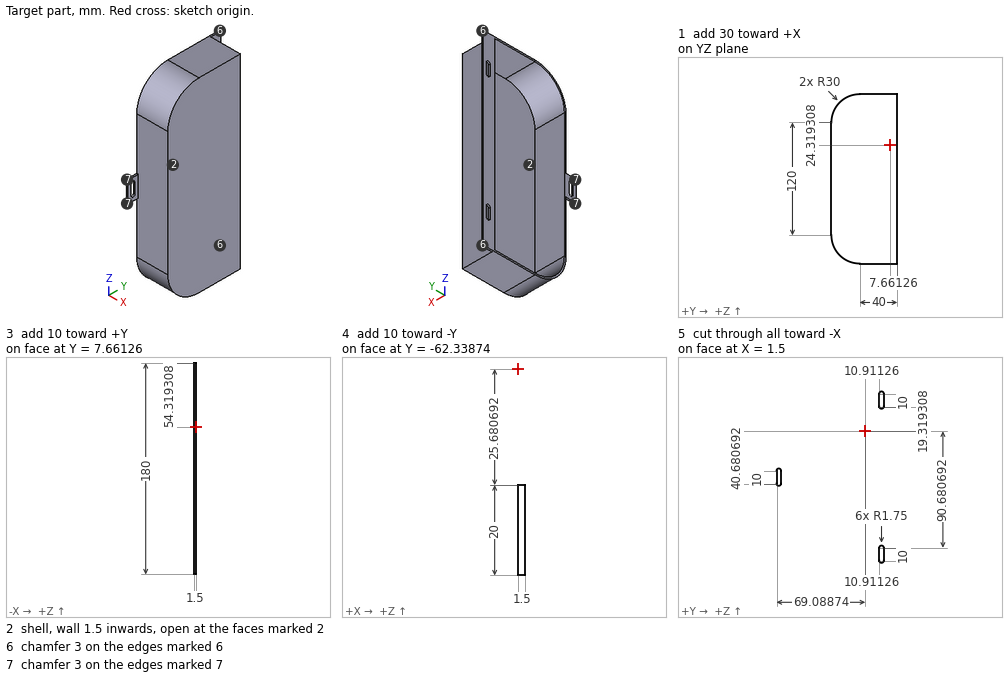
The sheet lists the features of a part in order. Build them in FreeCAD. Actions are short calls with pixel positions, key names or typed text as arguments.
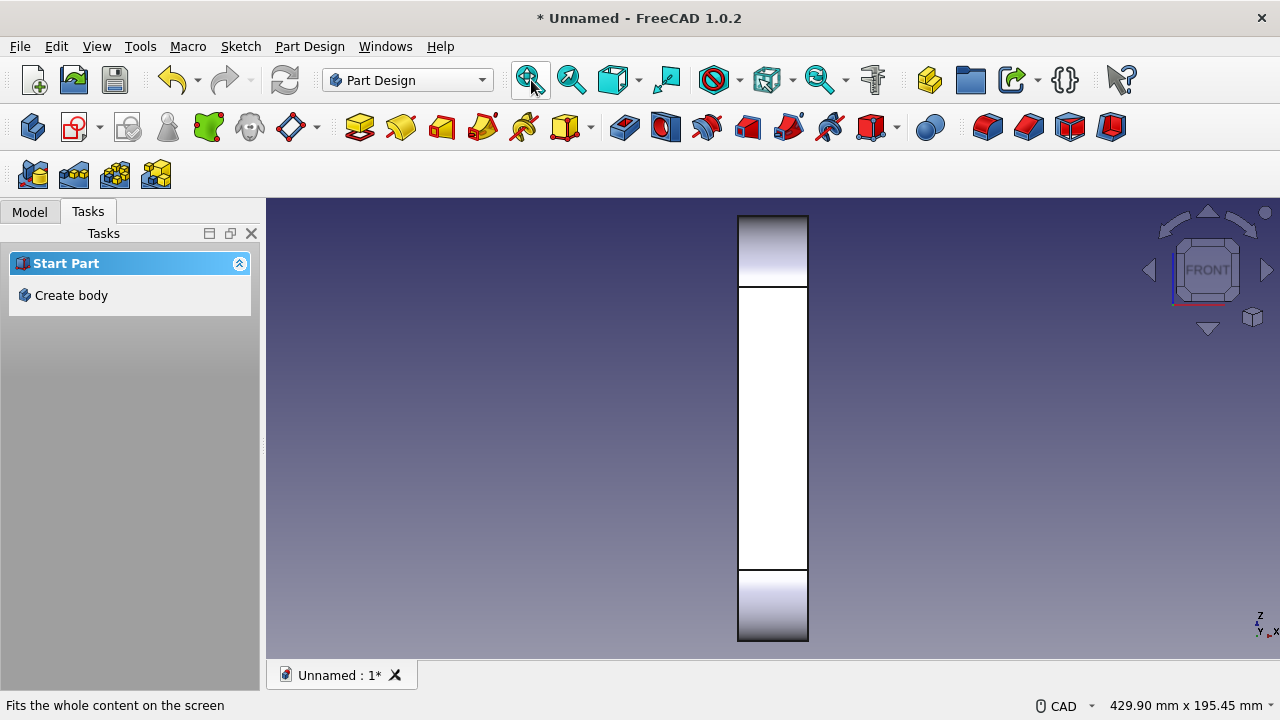
key(3)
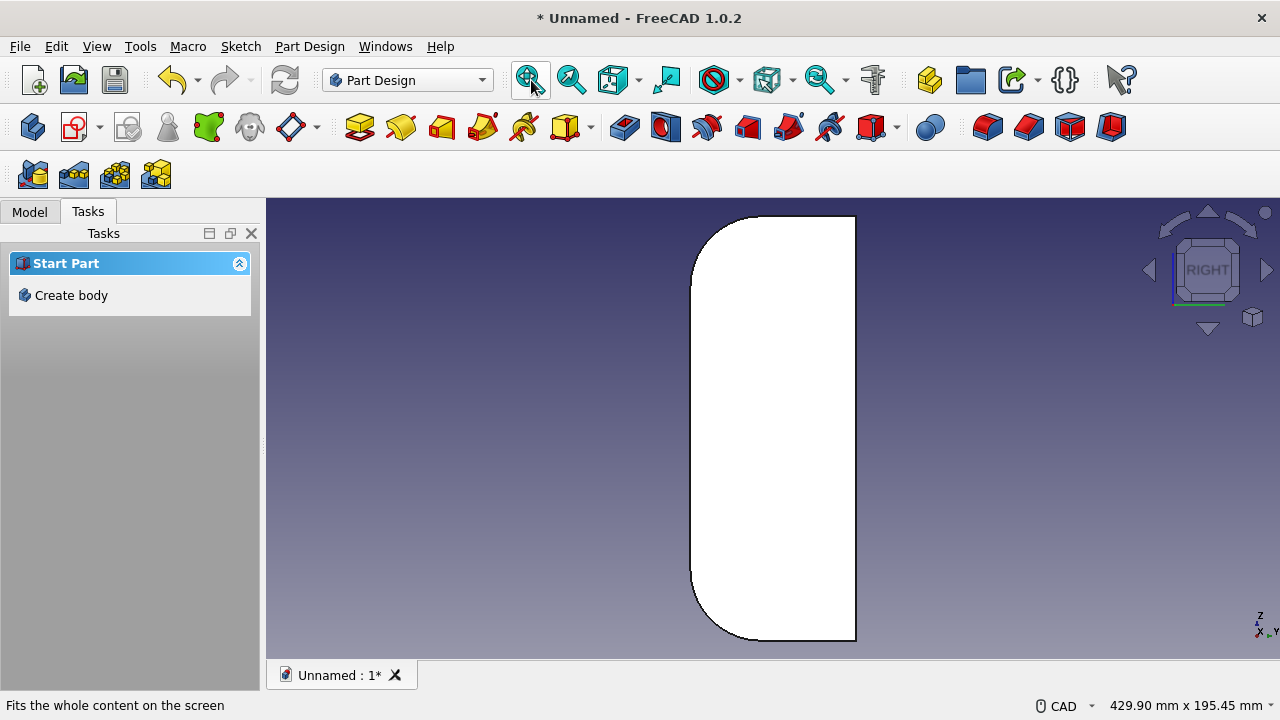
key(5)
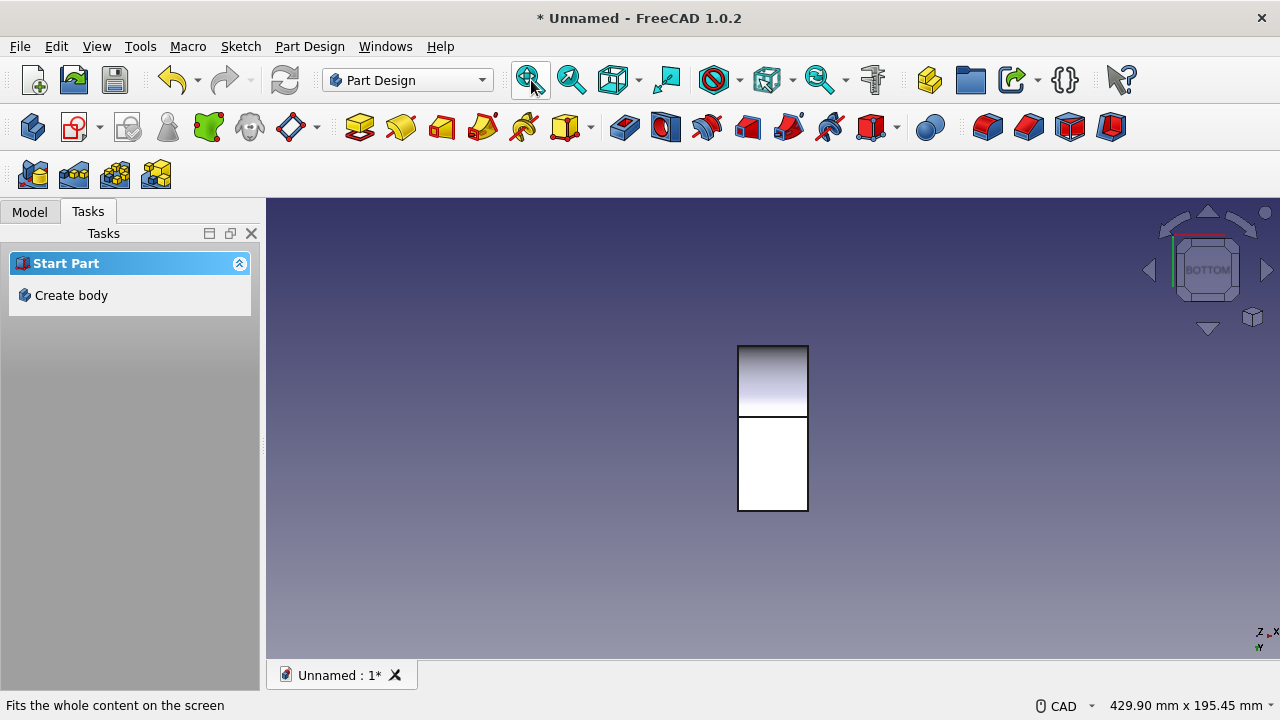
click(531, 80)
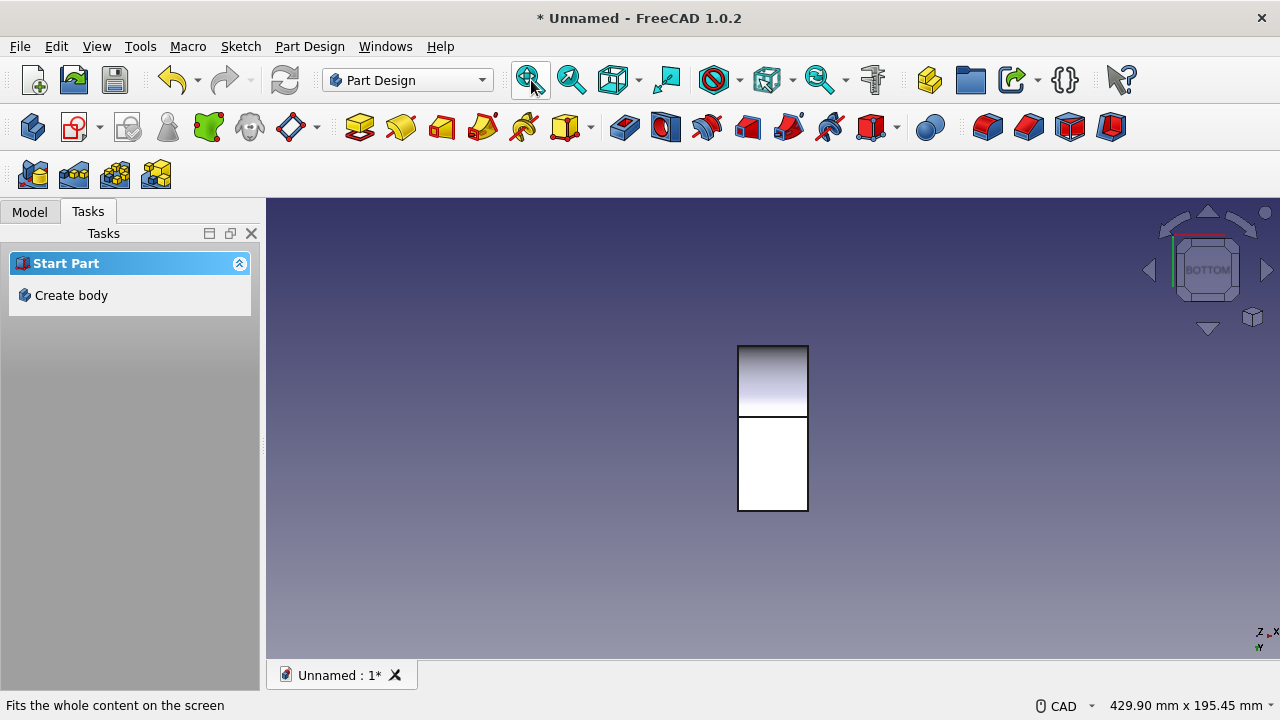
key(4)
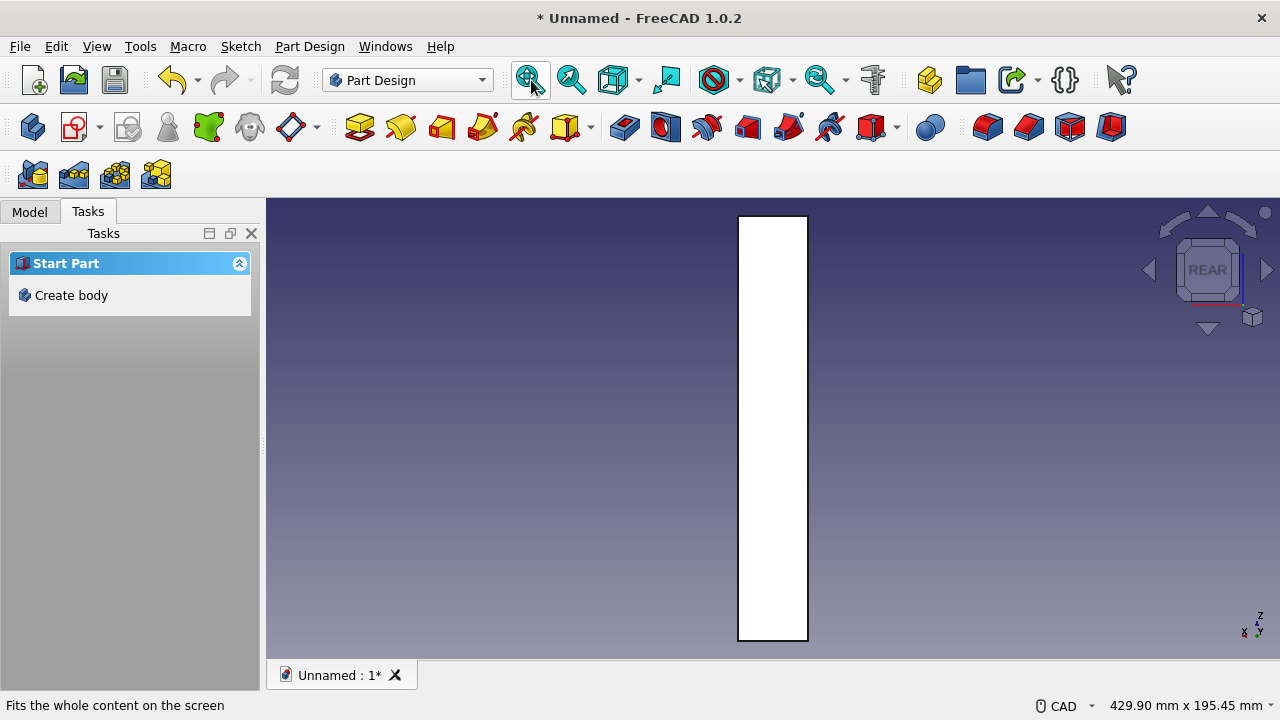
key(6)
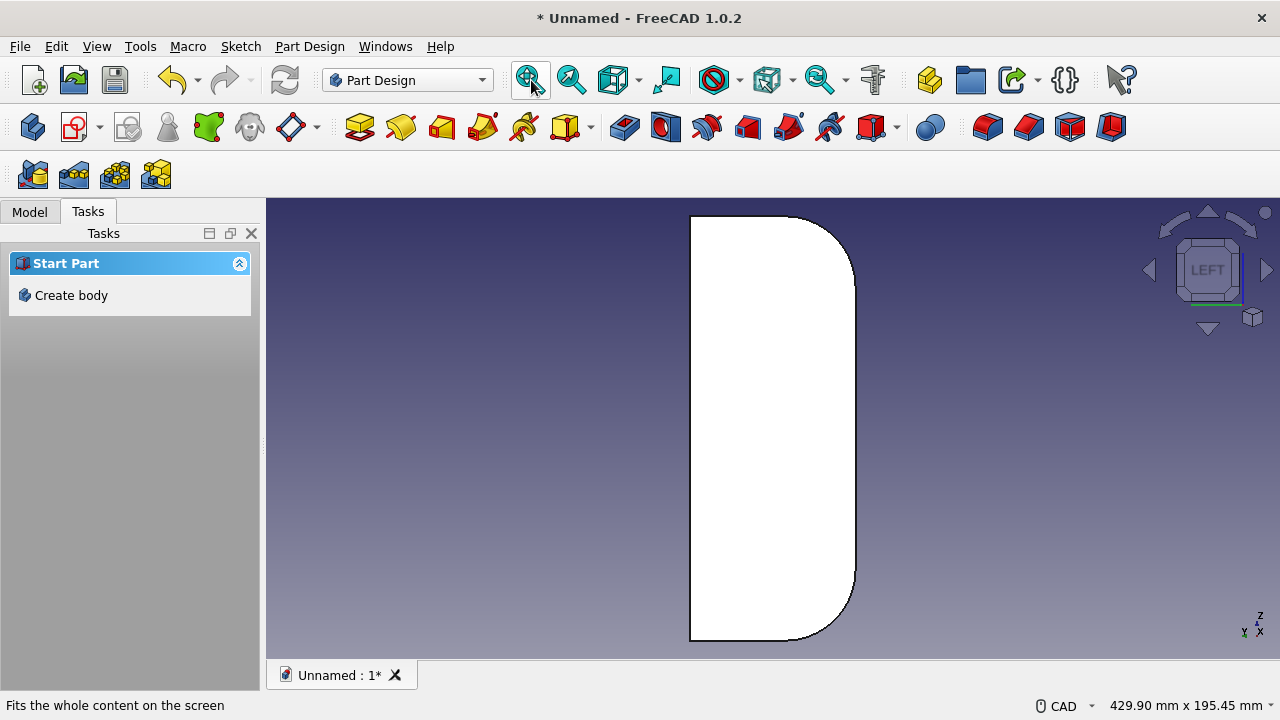
click(773, 549)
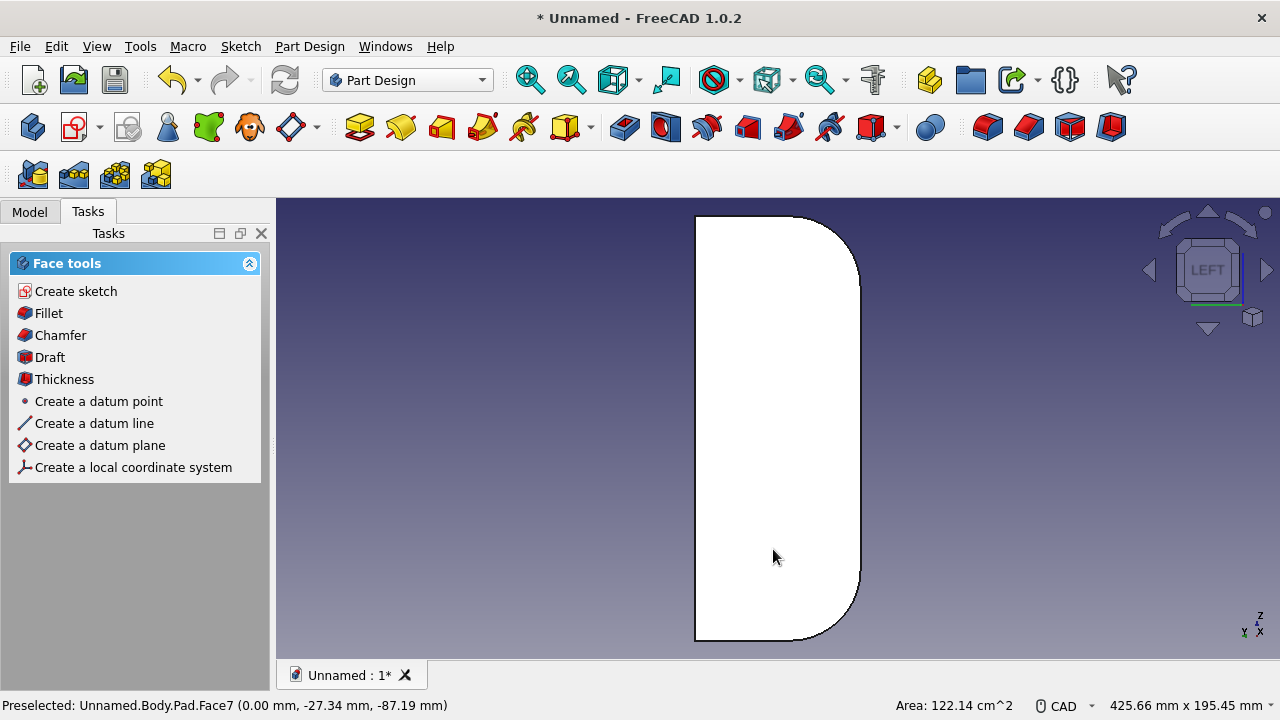
click(1111, 128)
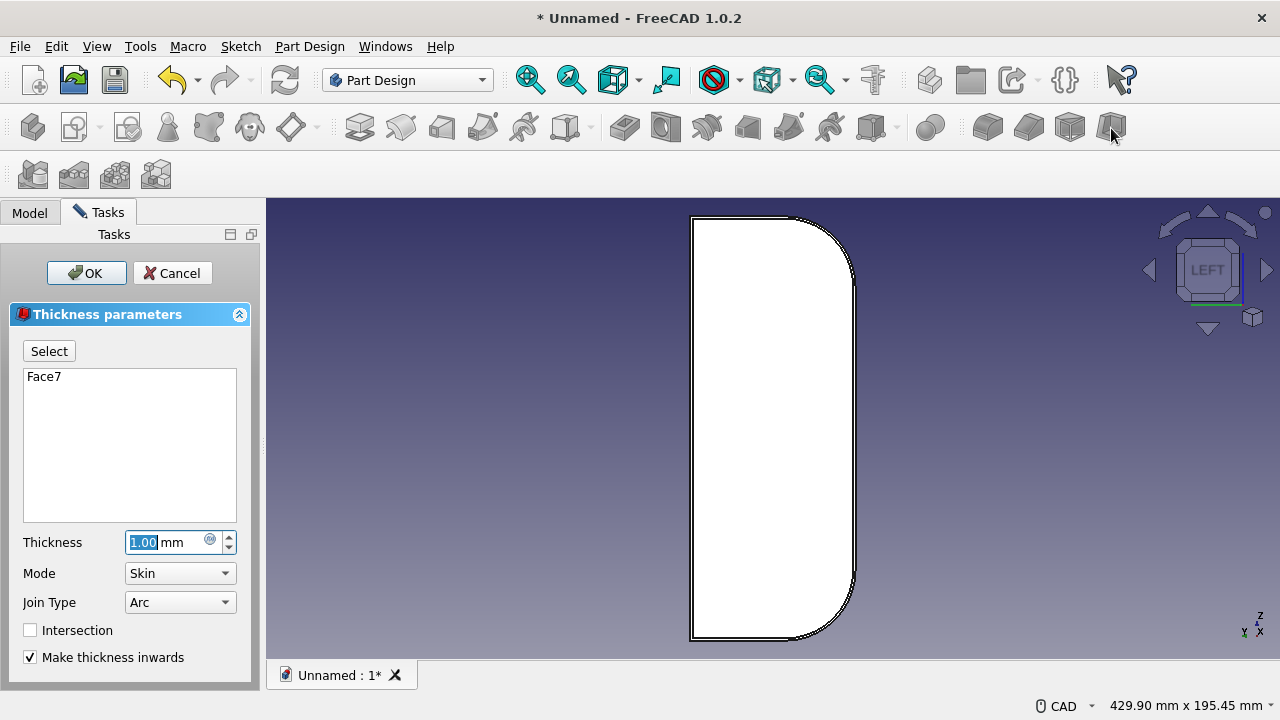
text(1.5)
key(Tab)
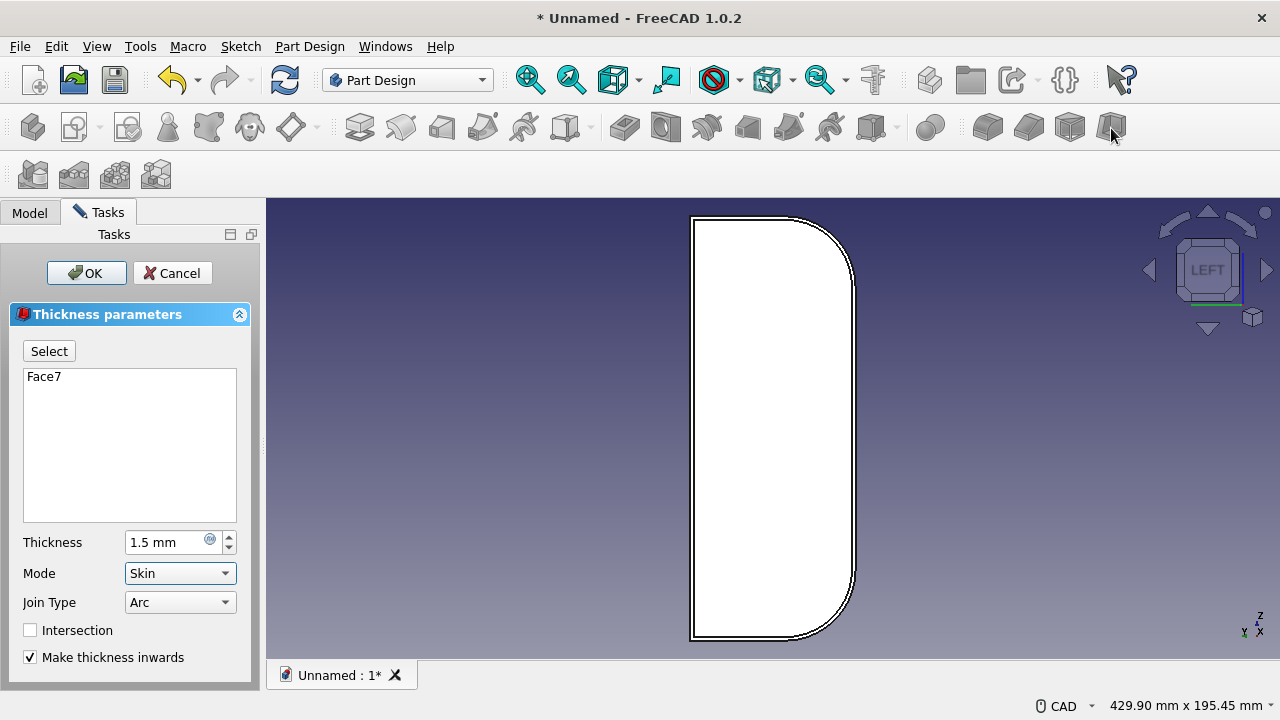
click(181, 602)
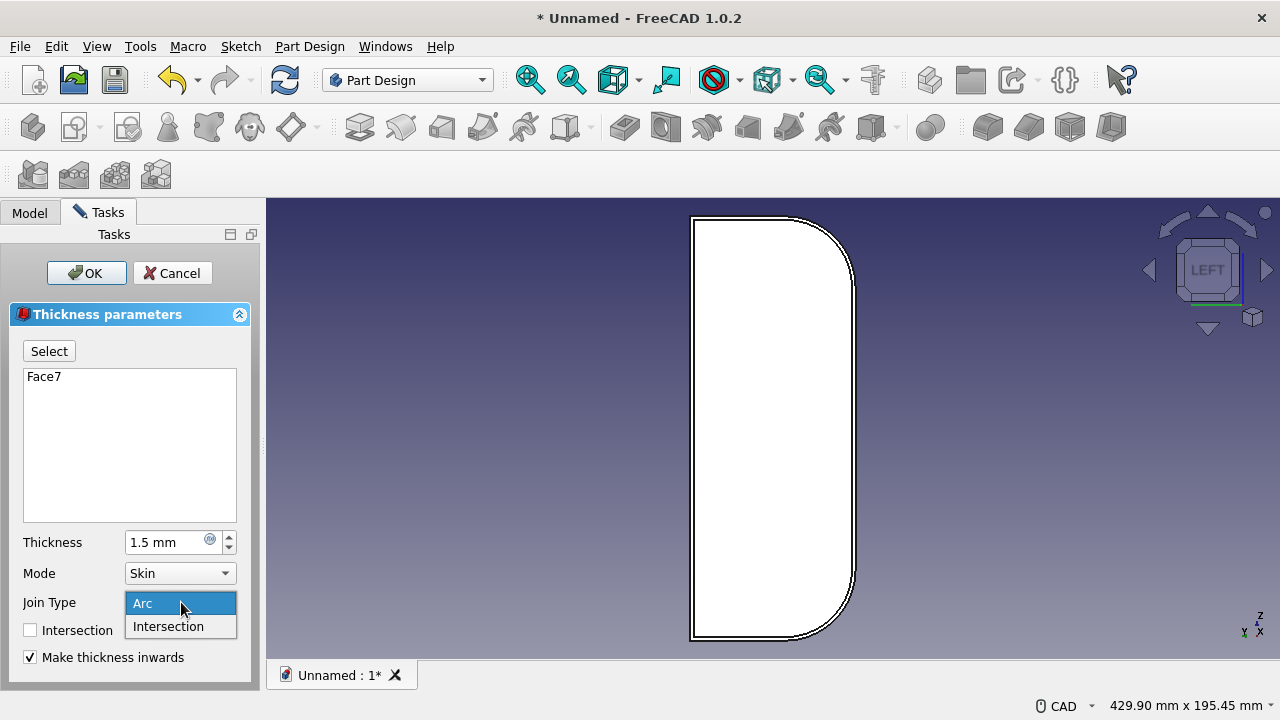
click(179, 626)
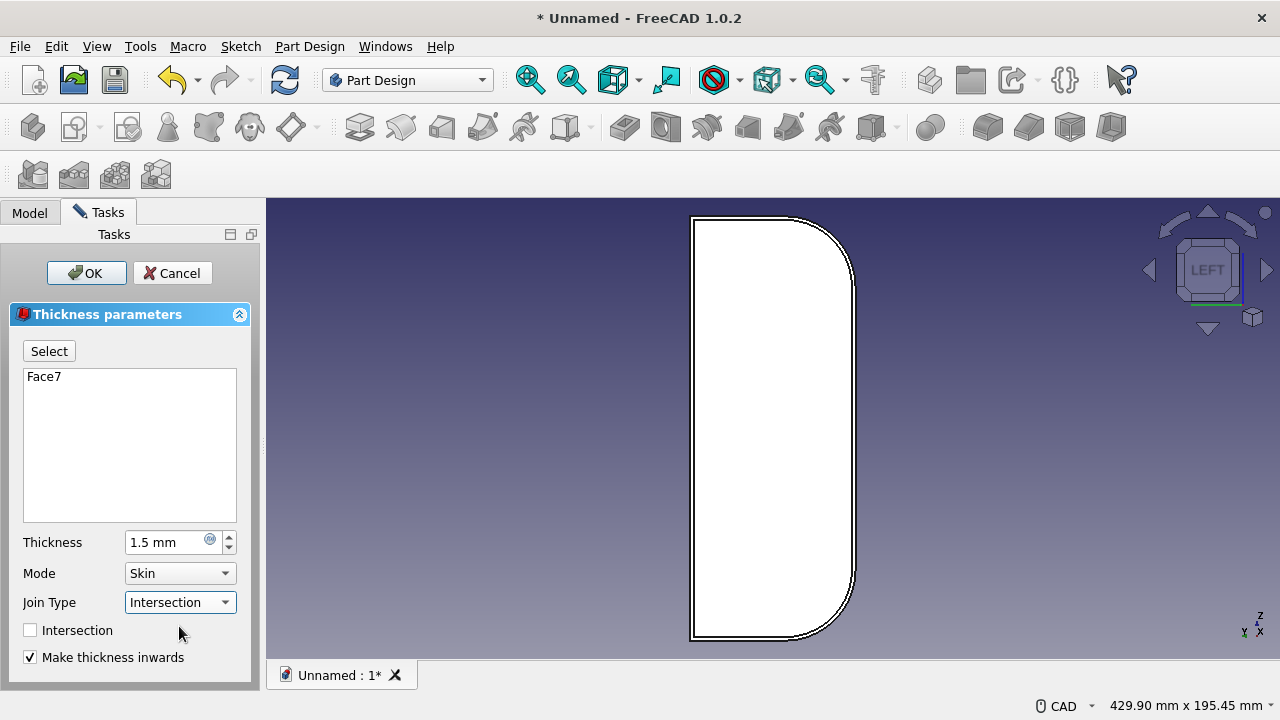
click(87, 273)